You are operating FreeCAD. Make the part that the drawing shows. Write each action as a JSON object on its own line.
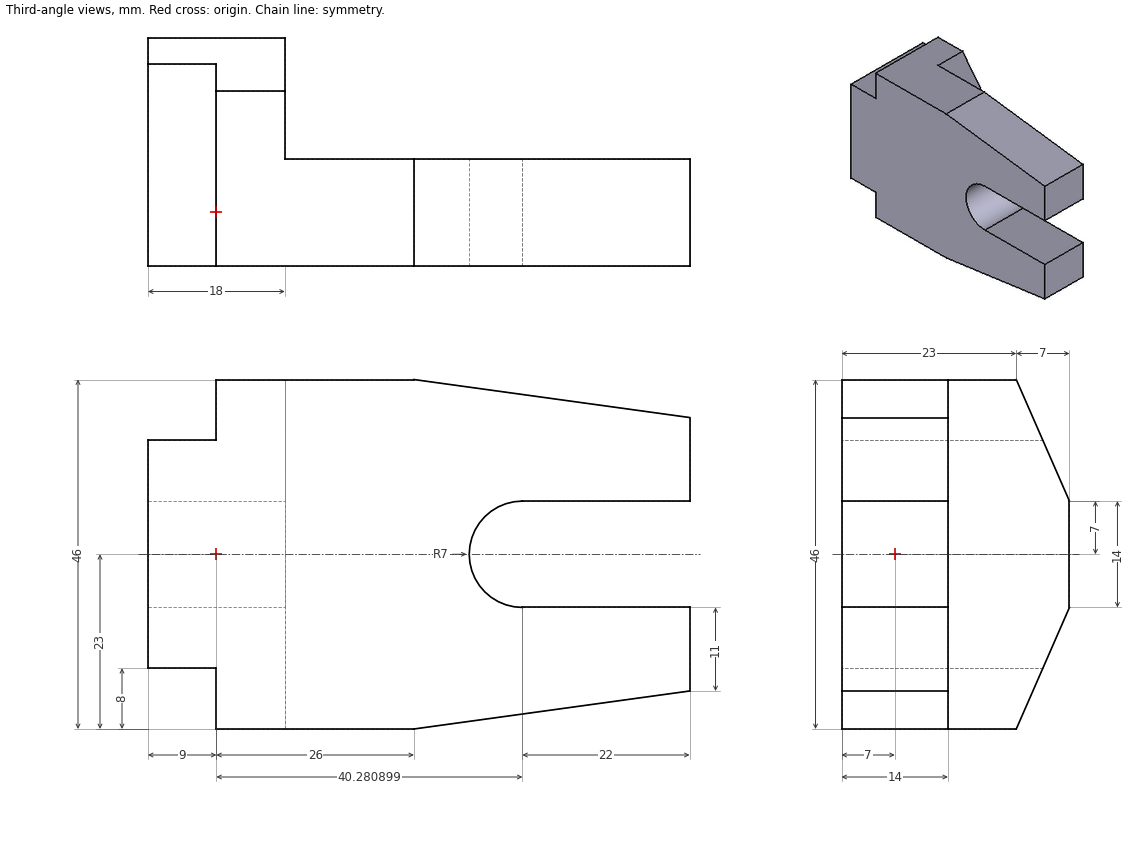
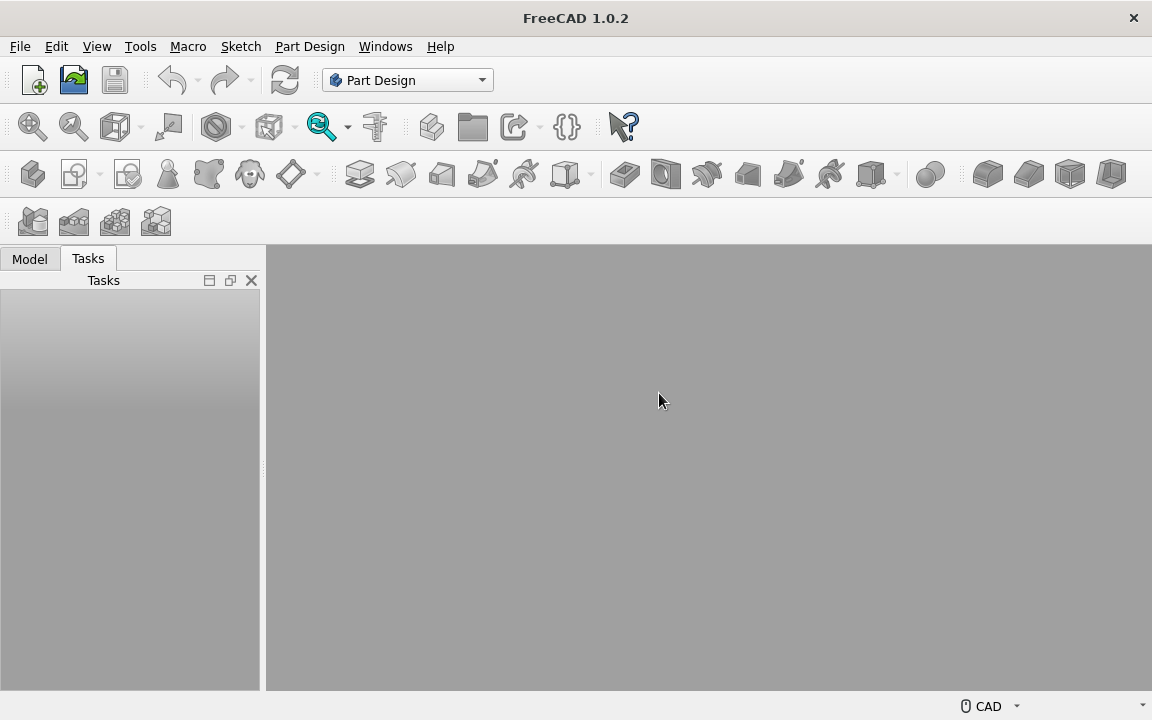
{"action": "key", "text": "ctrl+n"}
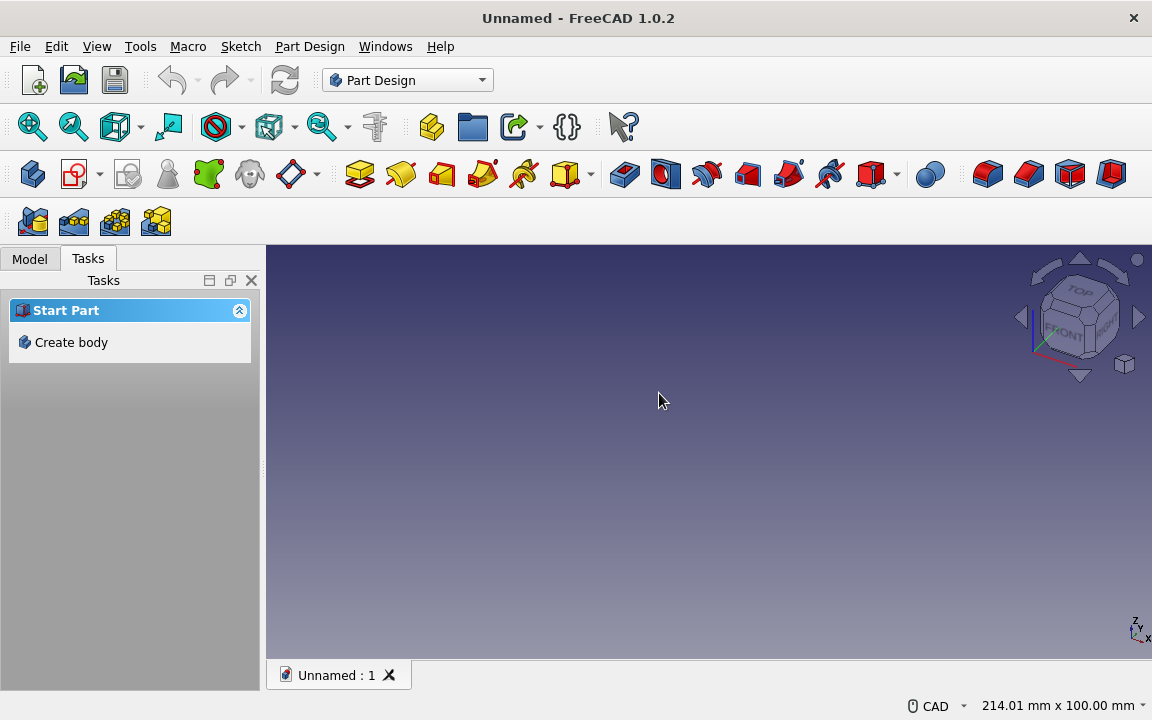
{"action": "left_click", "coordinate": [74, 174]}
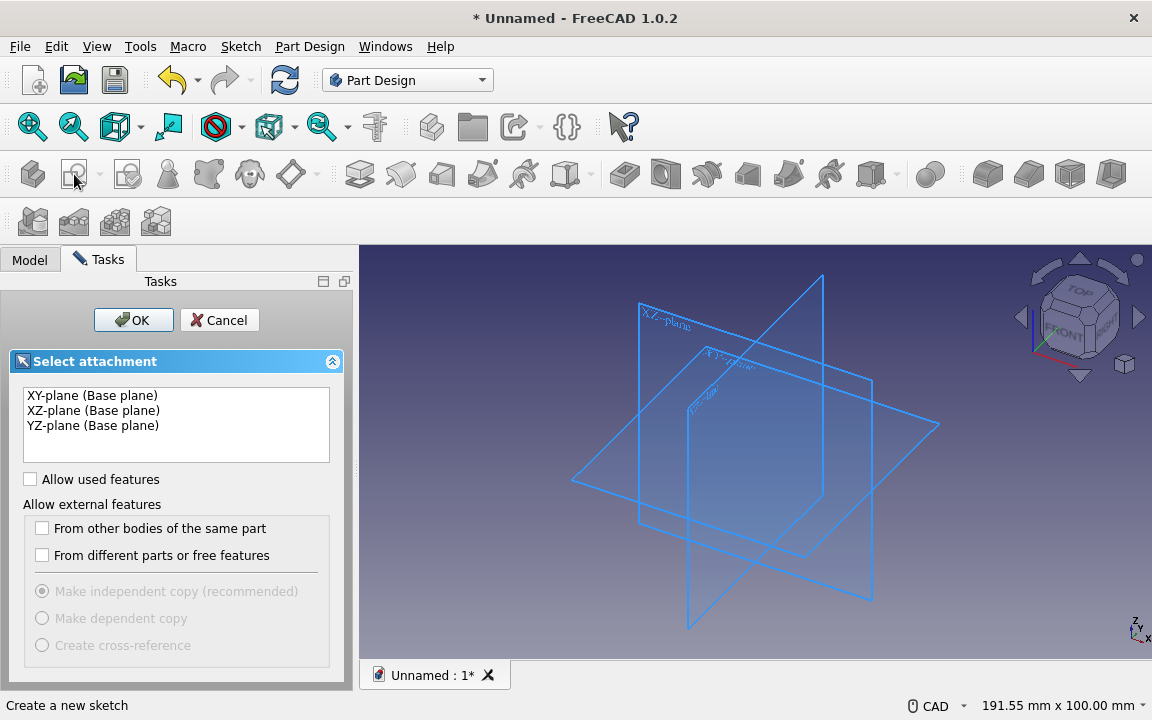
{"action": "left_click", "coordinate": [84, 410]}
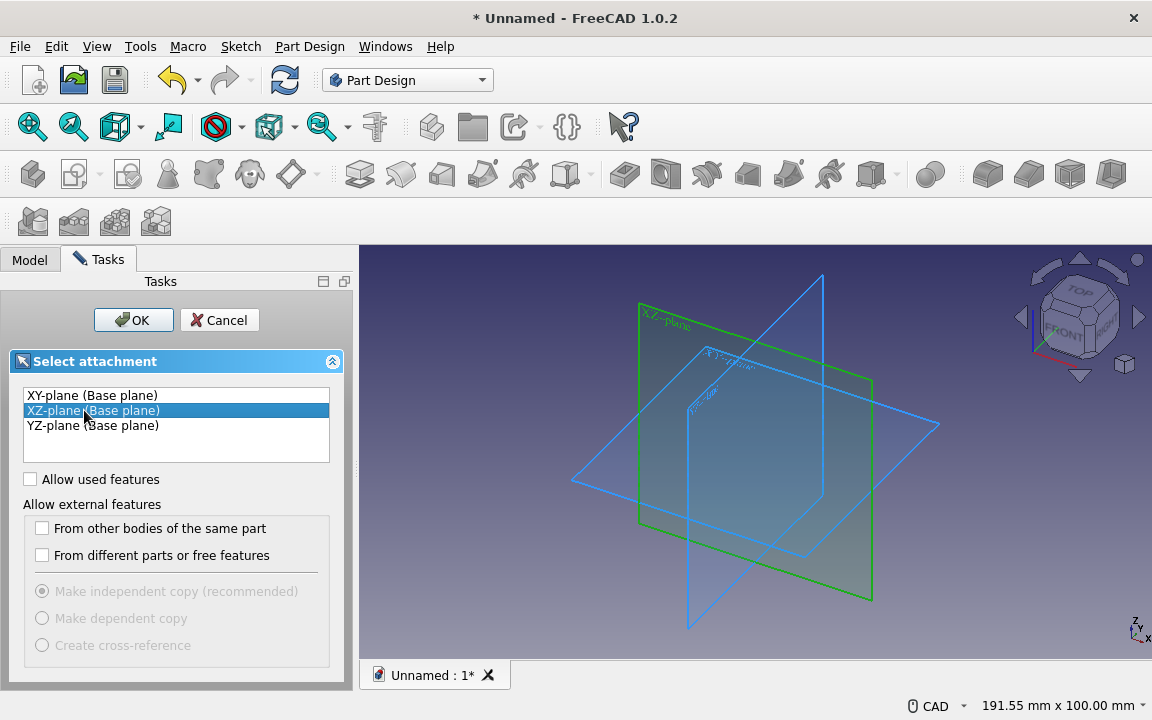
{"action": "left_click", "coordinate": [134, 320]}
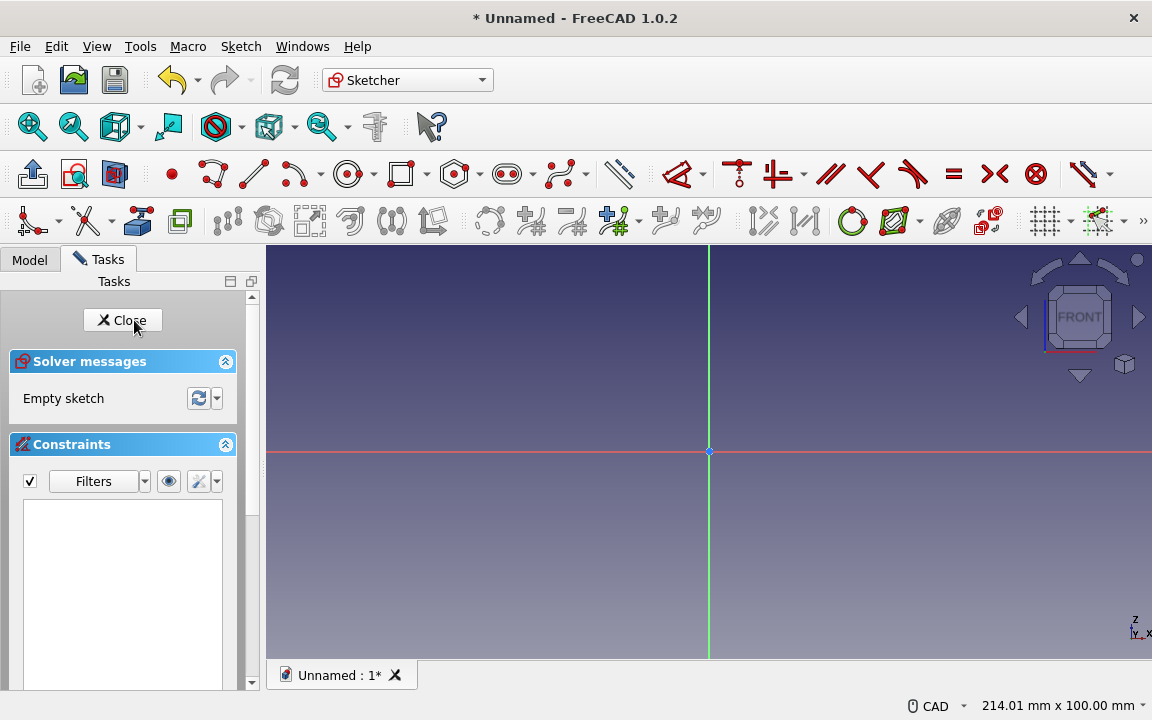
{"action": "scroll", "coordinate": [294, 452], "scroll_direction": "down", "scroll_amount": 1}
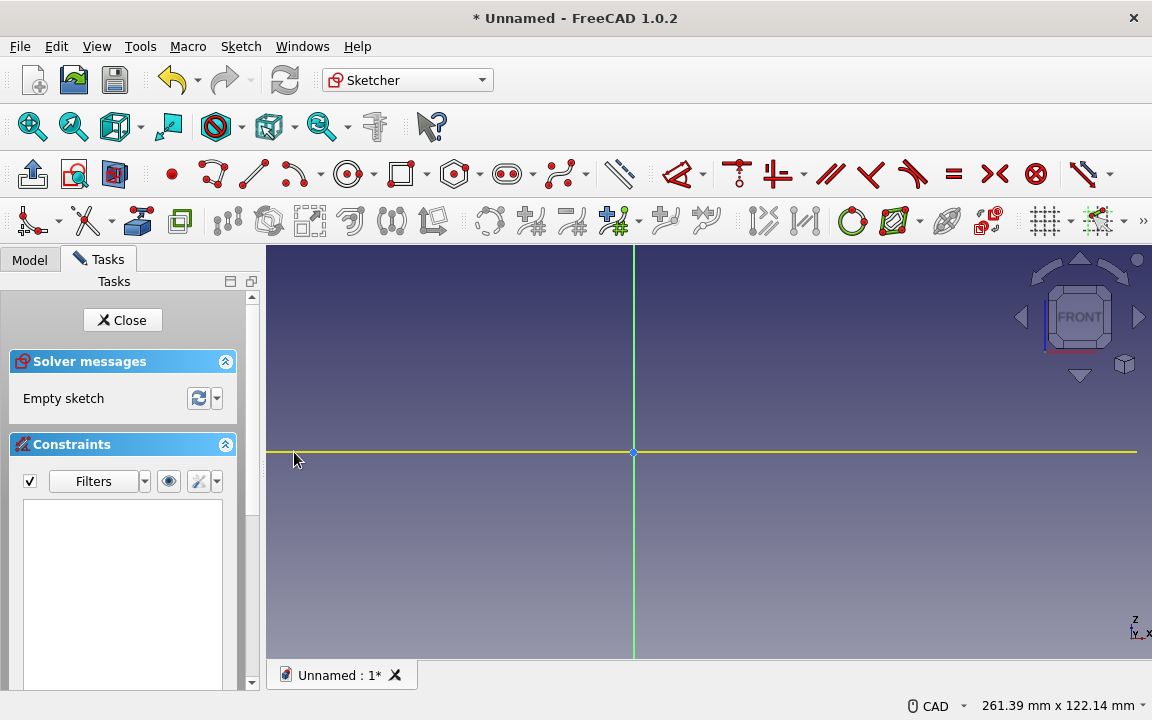
{"action": "scroll", "coordinate": [940, 452], "scroll_direction": "up", "scroll_amount": 2}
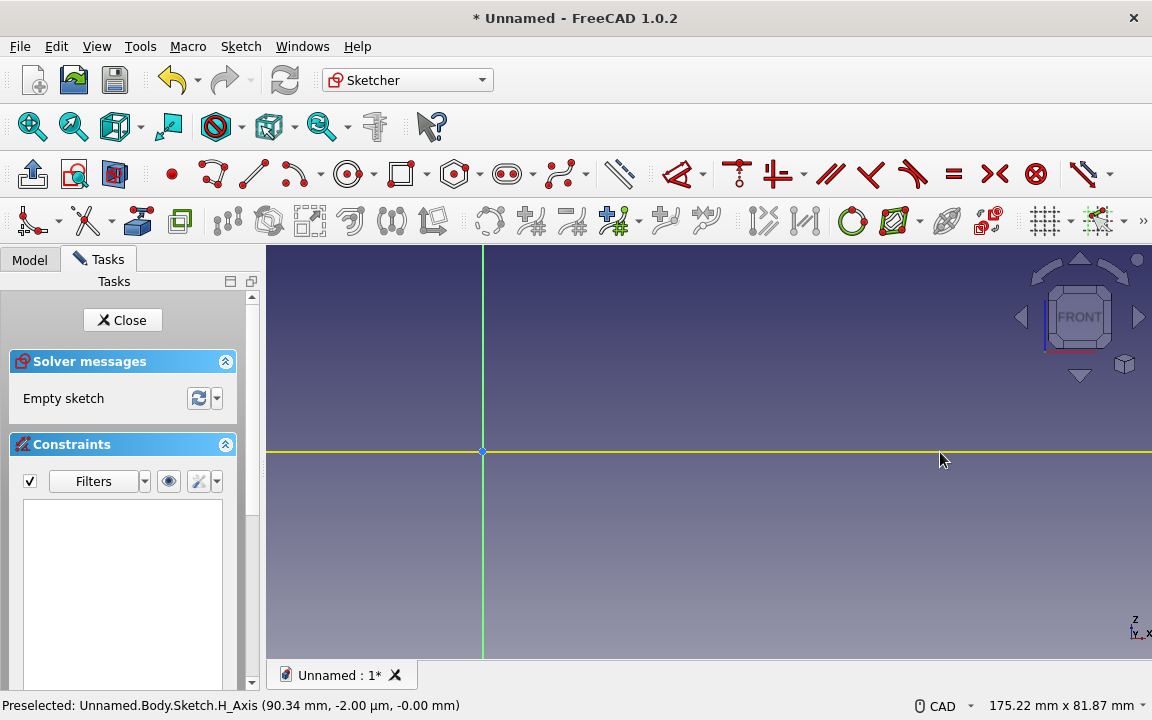
{"action": "left_click", "coordinate": [213, 174]}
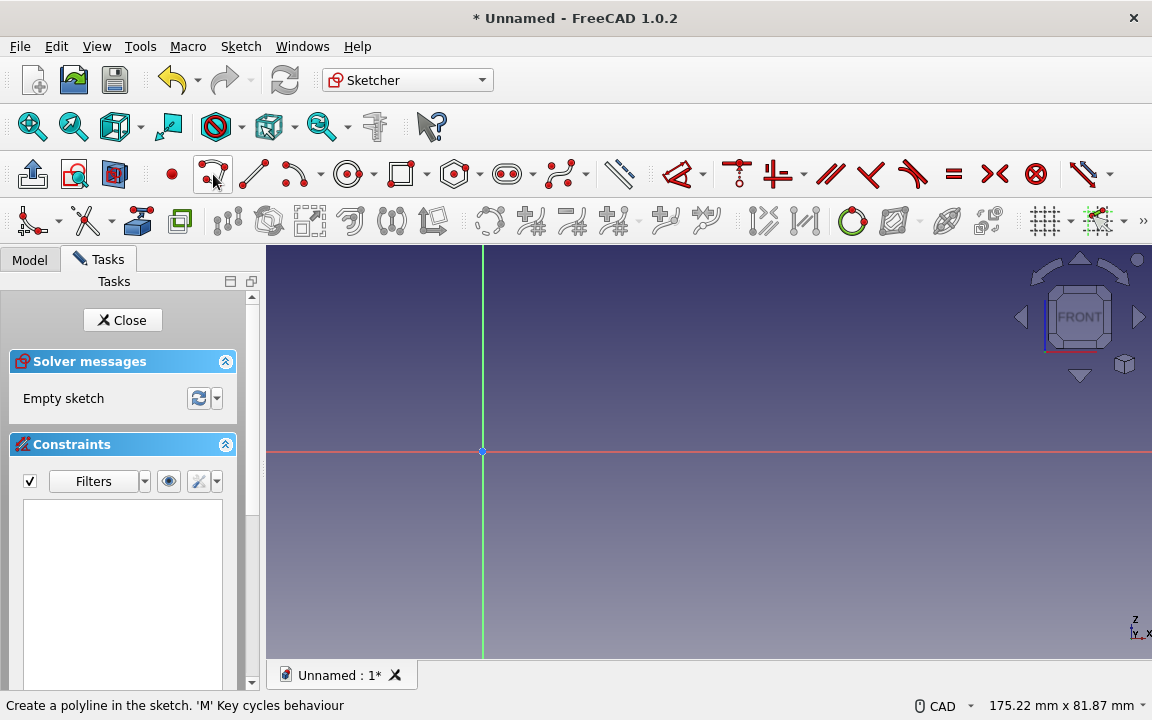
{"action": "left_click", "coordinate": [686, 487]}
{"action": "left_click", "coordinate": [798, 487]}
{"action": "left_click", "coordinate": [798, 543]}
{"action": "left_click", "coordinate": [614, 568]}
{"action": "left_click", "coordinate": [483, 568]}
{"action": "left_click", "coordinate": [492, 336]}
{"action": "left_click", "coordinate": [614, 336]}
{"action": "left_click", "coordinate": [798, 361]}
{"action": "left_click", "coordinate": [798, 416]}
{"action": "left_click", "coordinate": [686, 416]}
{"action": "right_click", "coordinate": [686, 416]}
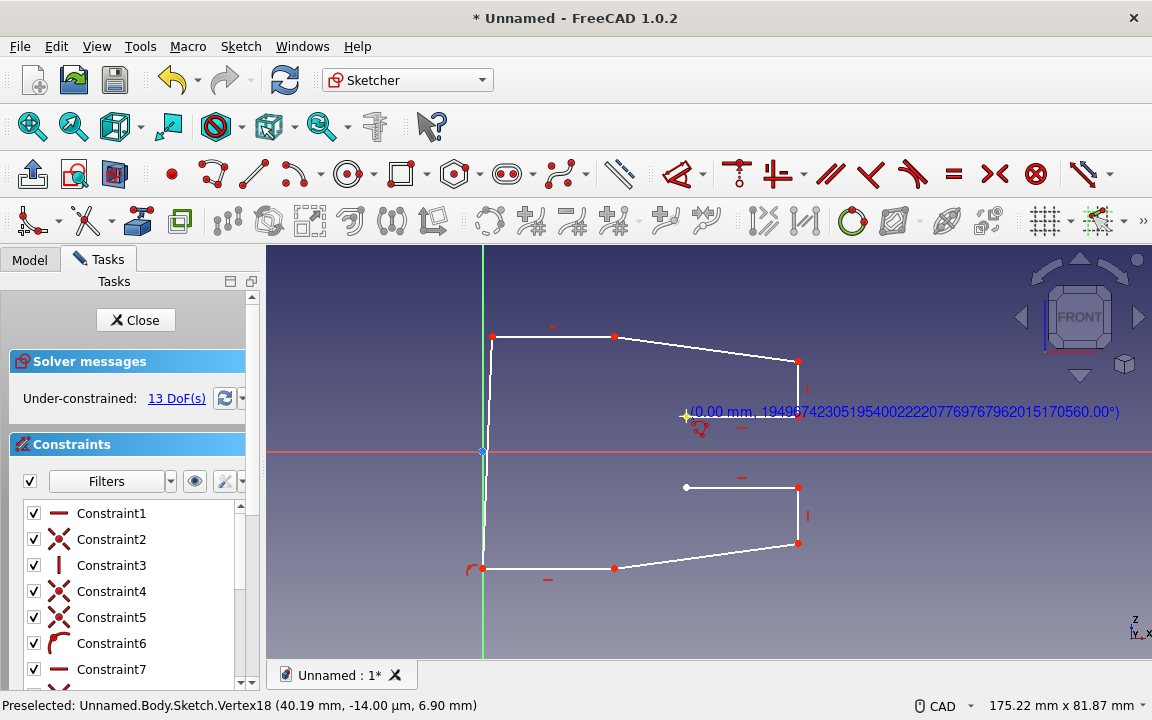
{"action": "key", "text": "g 3 a"}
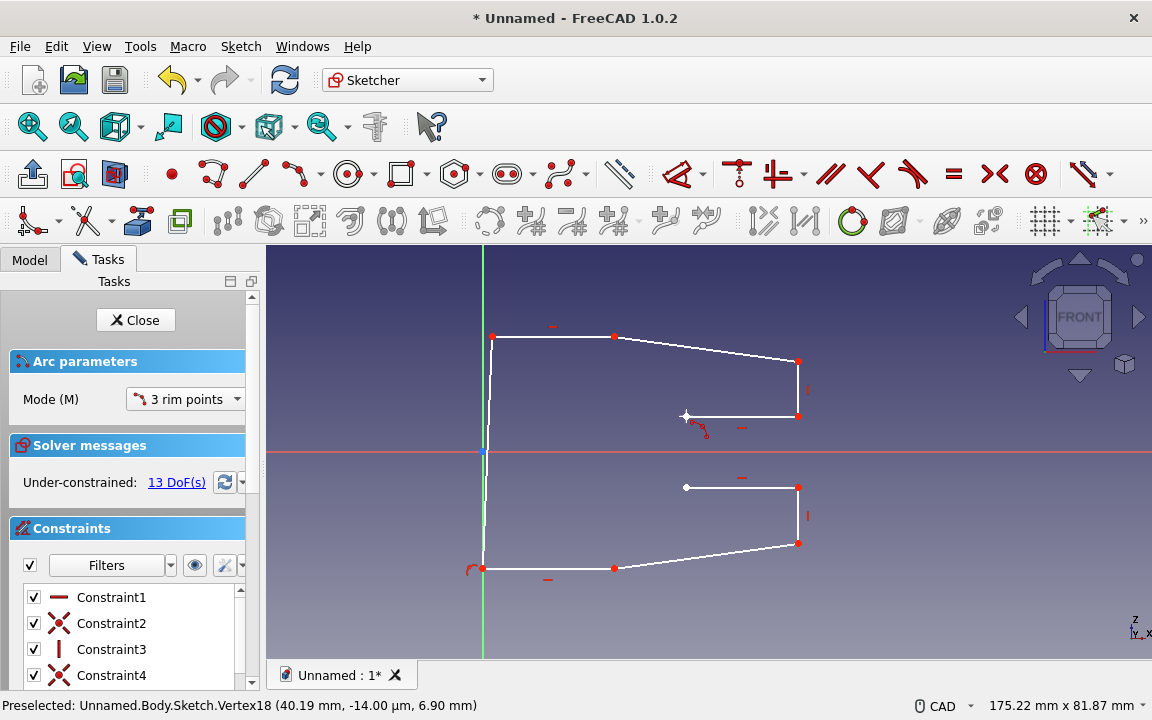
{"action": "left_click", "coordinate": [686, 417]}
{"action": "left_click", "coordinate": [686, 488]}
{"action": "left_click", "coordinate": [658, 431]}
{"action": "key", "text": "Escape"}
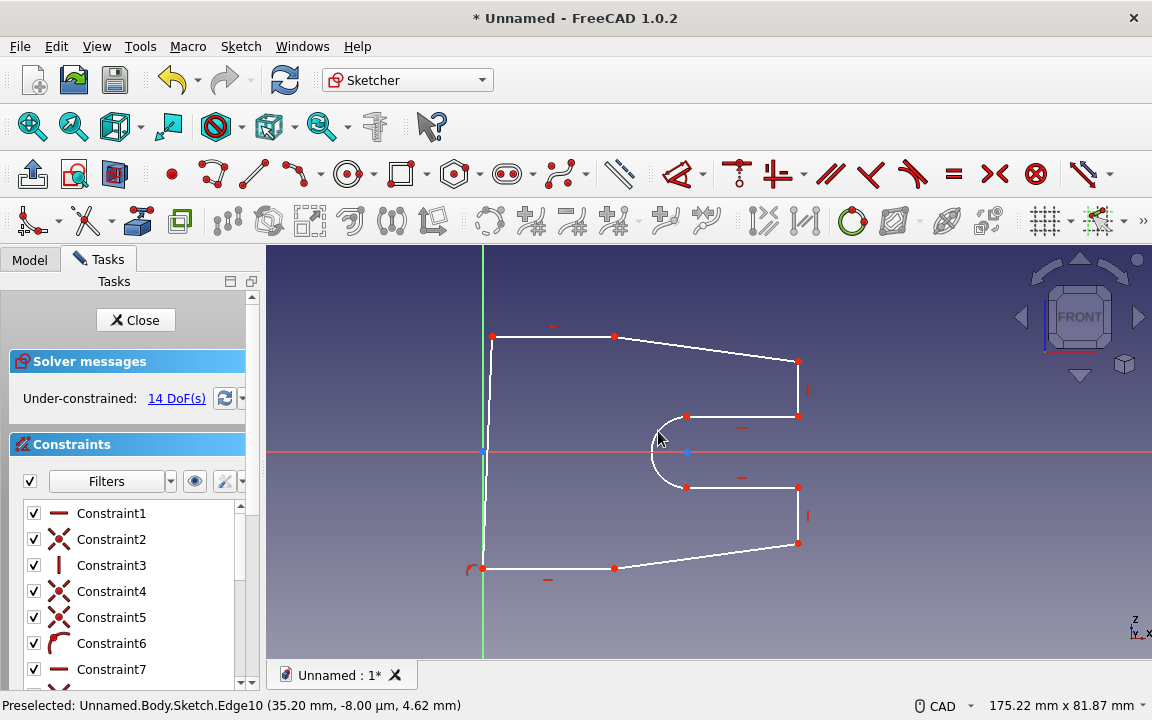
{"action": "left_click", "coordinate": [720, 488]}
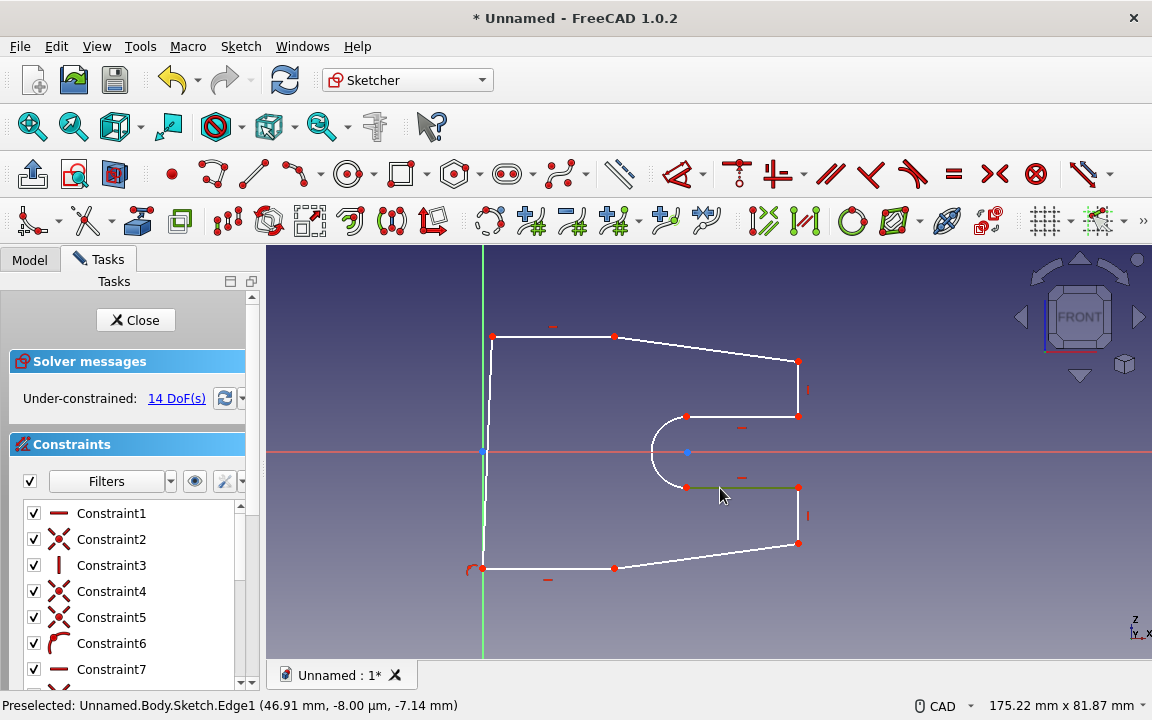
{"action": "left_click", "coordinate": [658, 432]}